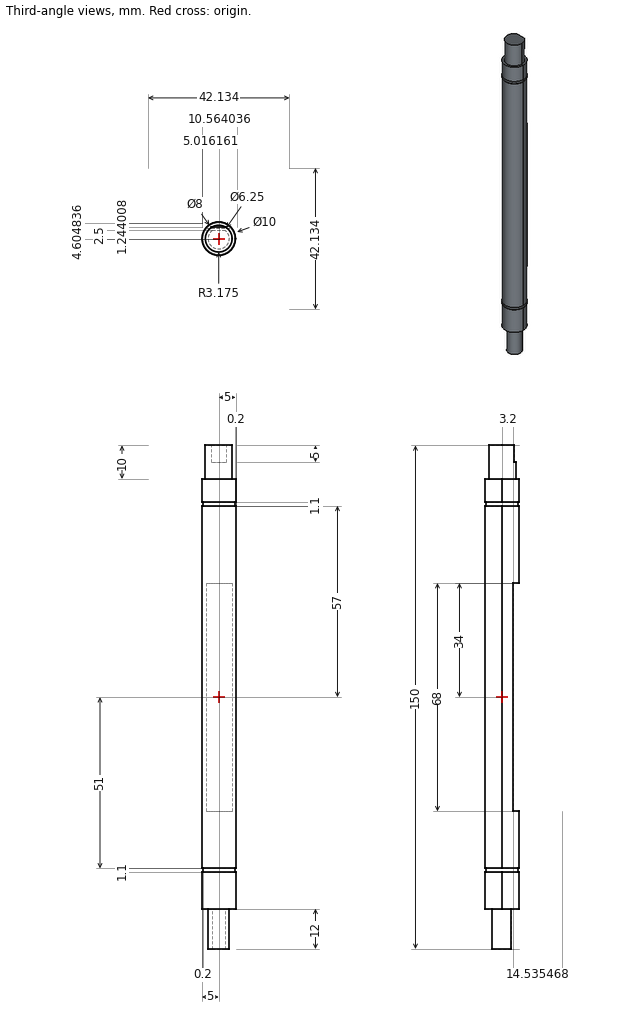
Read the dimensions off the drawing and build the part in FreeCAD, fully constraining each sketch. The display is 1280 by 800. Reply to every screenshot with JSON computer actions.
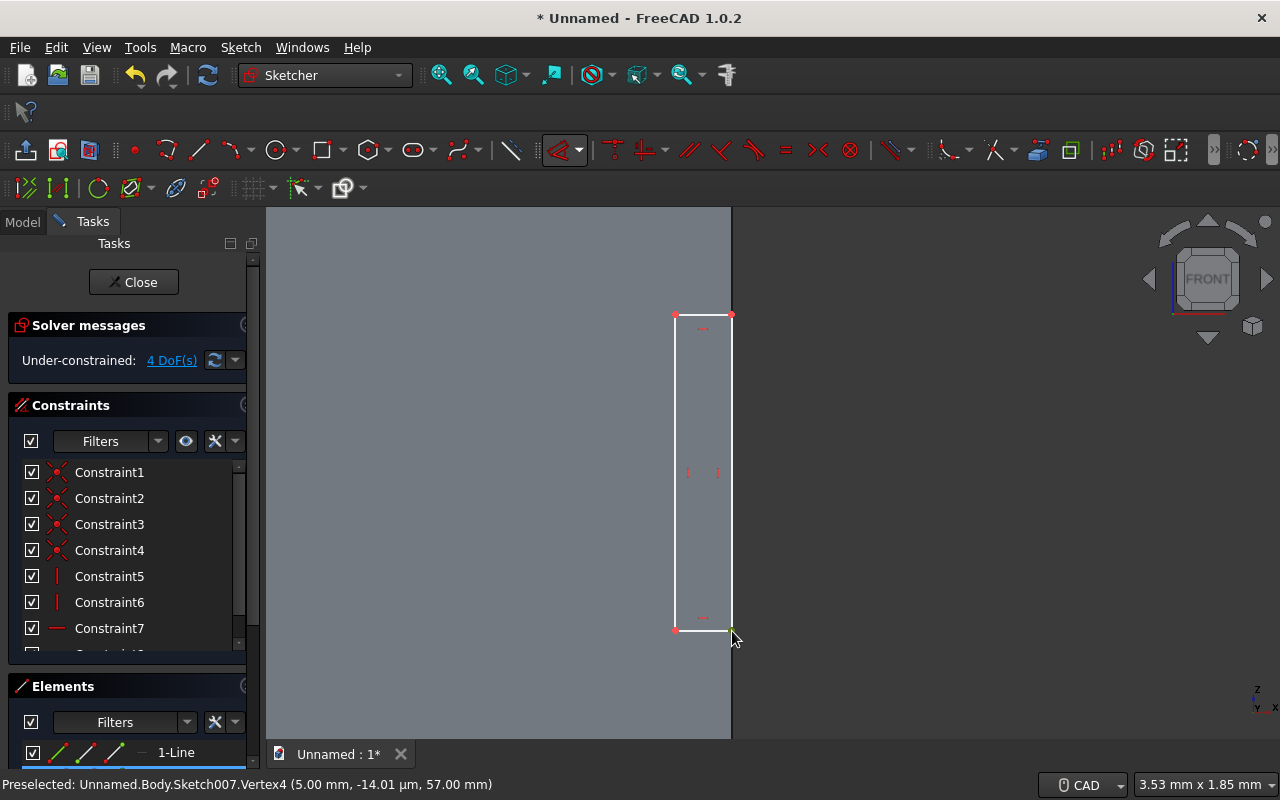
{"action": "key", "text": "l"}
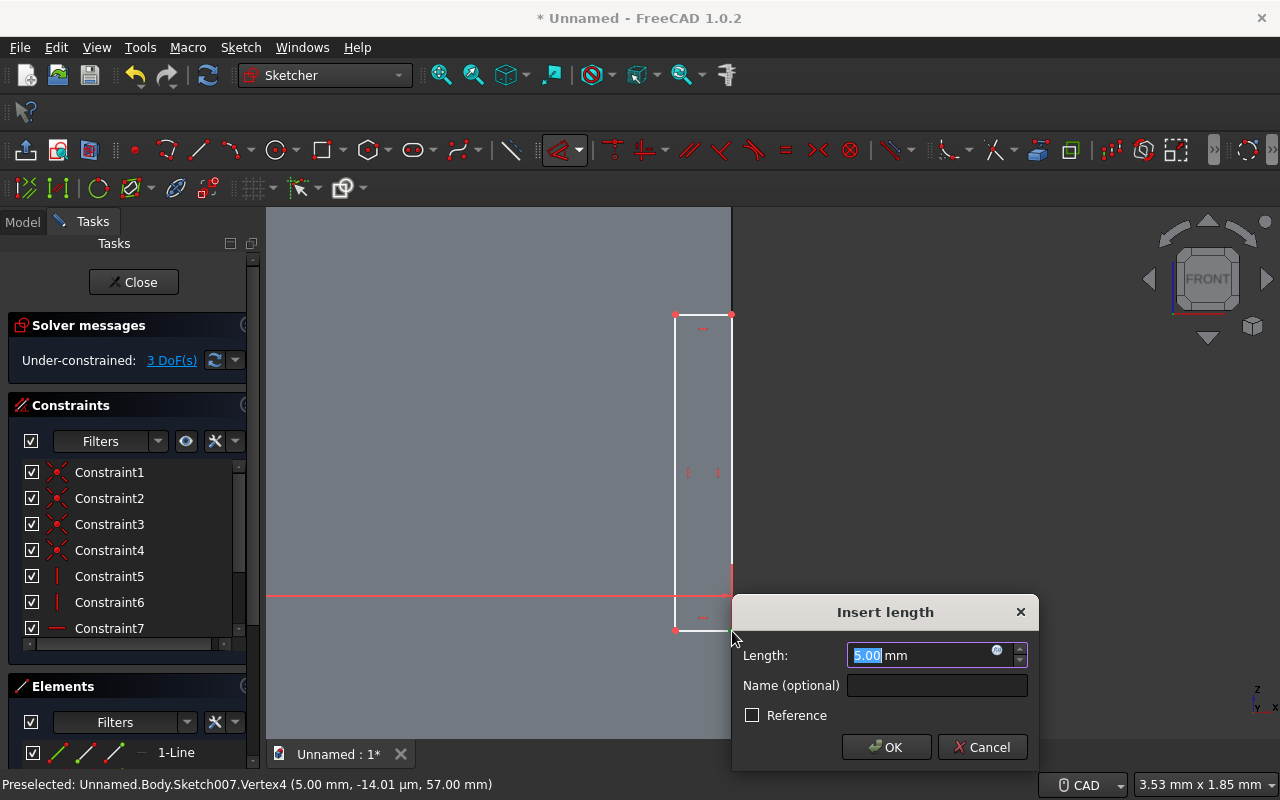
{"action": "type", "text": "5"}
{"action": "key", "text": "Return"}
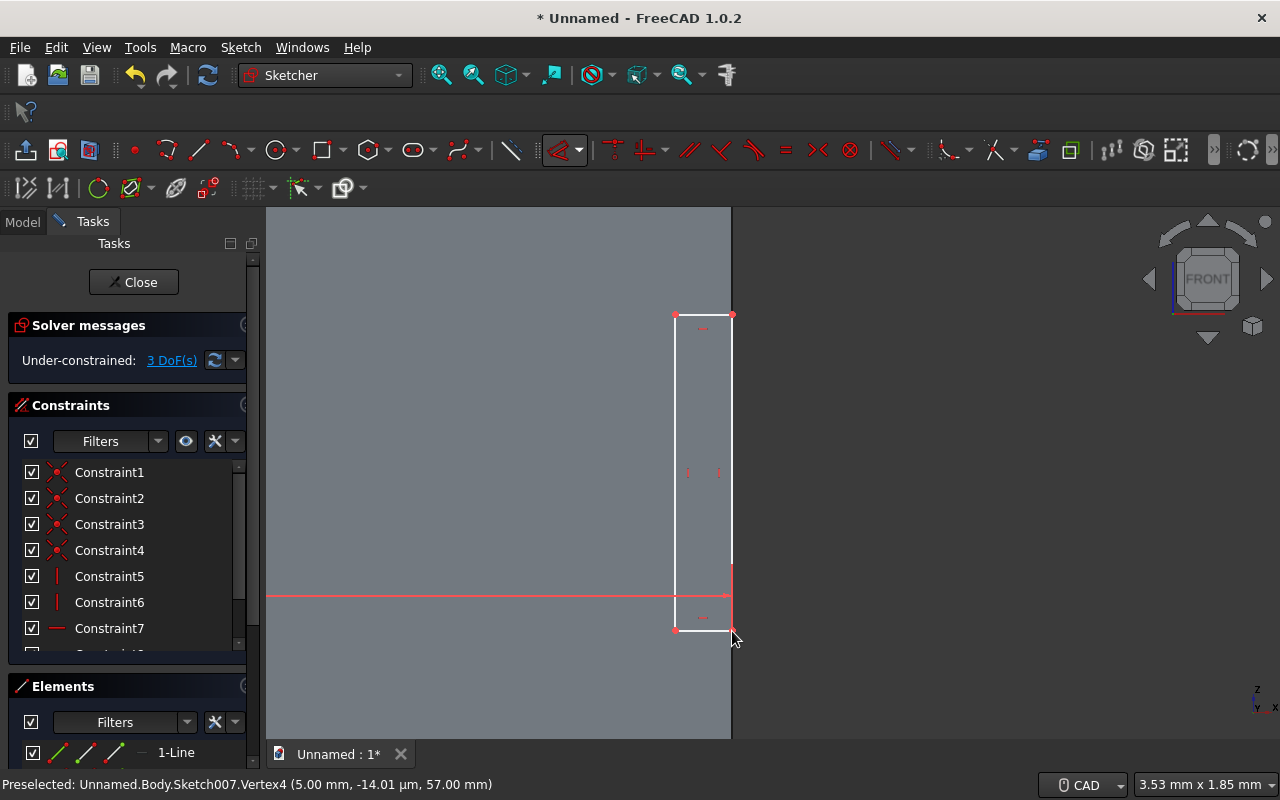
{"action": "left_click", "coordinate": [675, 410]}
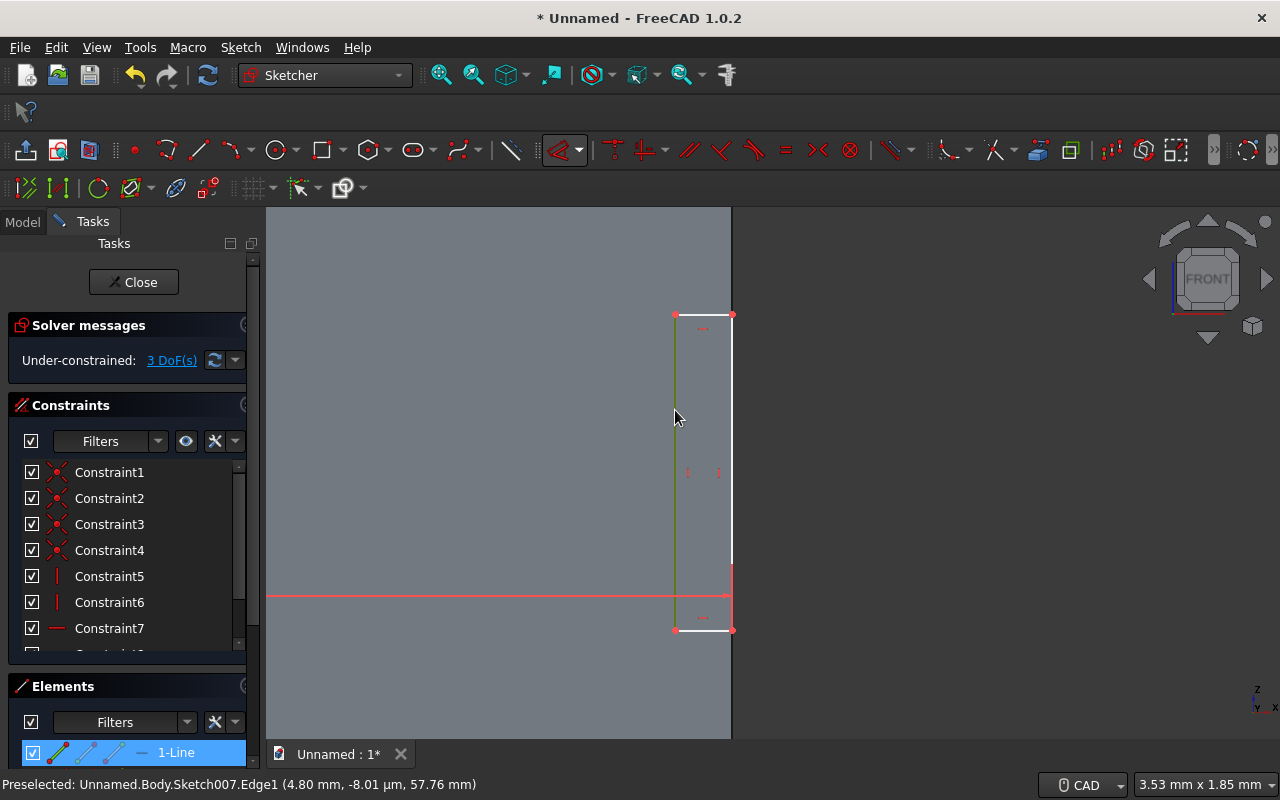
{"action": "key", "text": "i"}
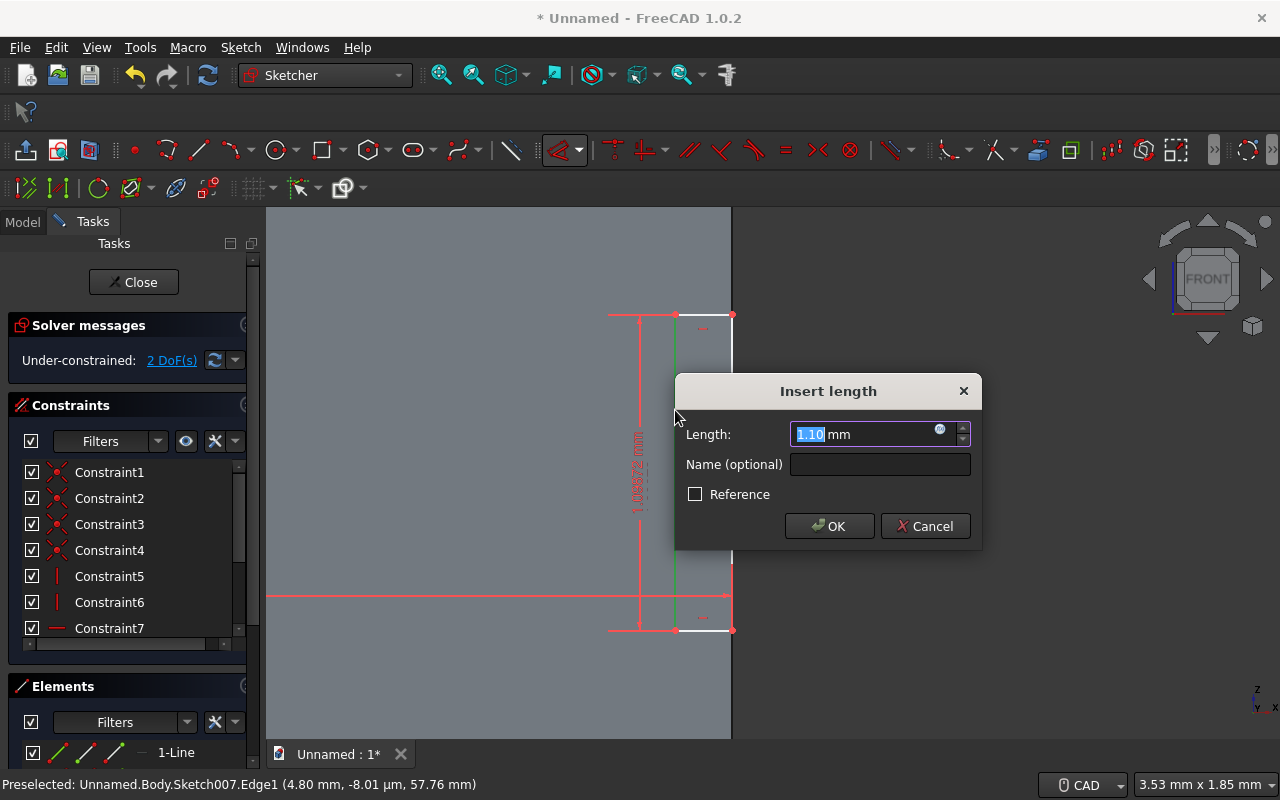
{"action": "type", "text": "1.1"}
{"action": "key", "text": "Return"}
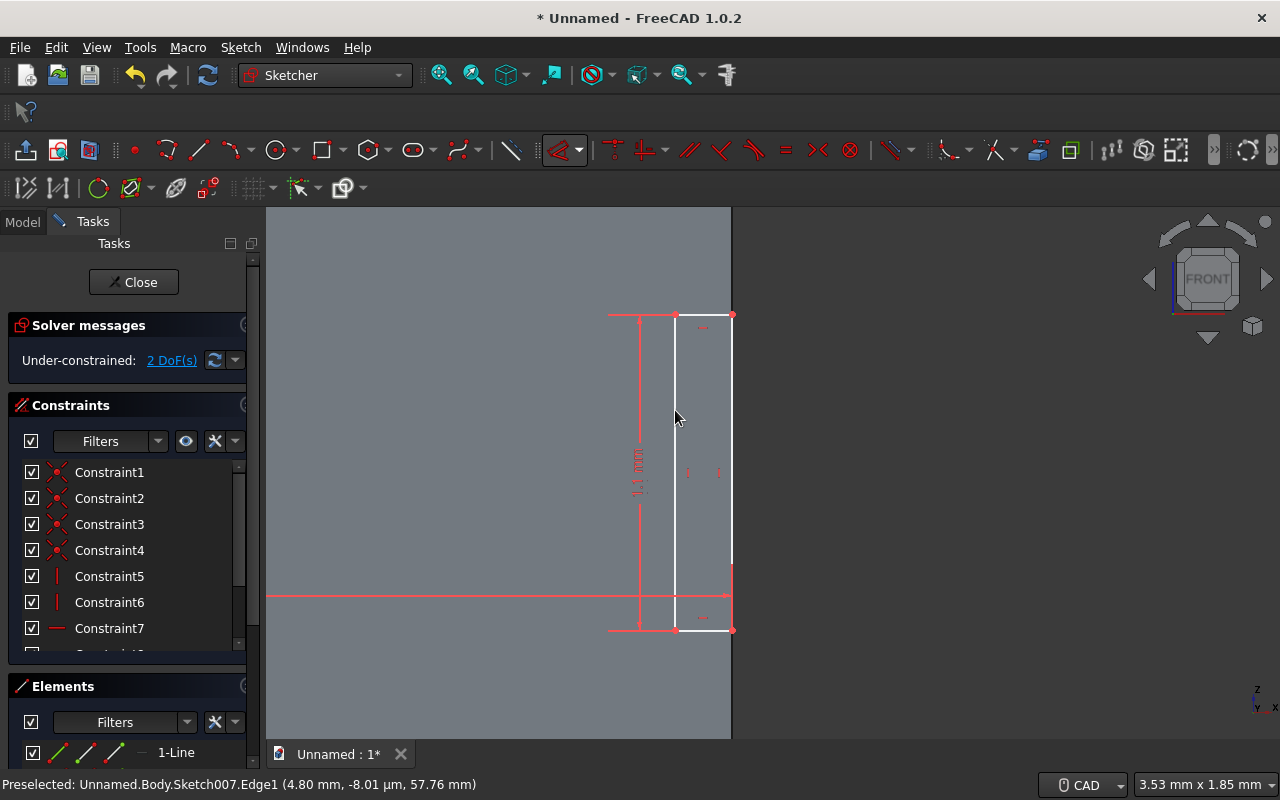
{"action": "left_click", "coordinate": [692, 631]}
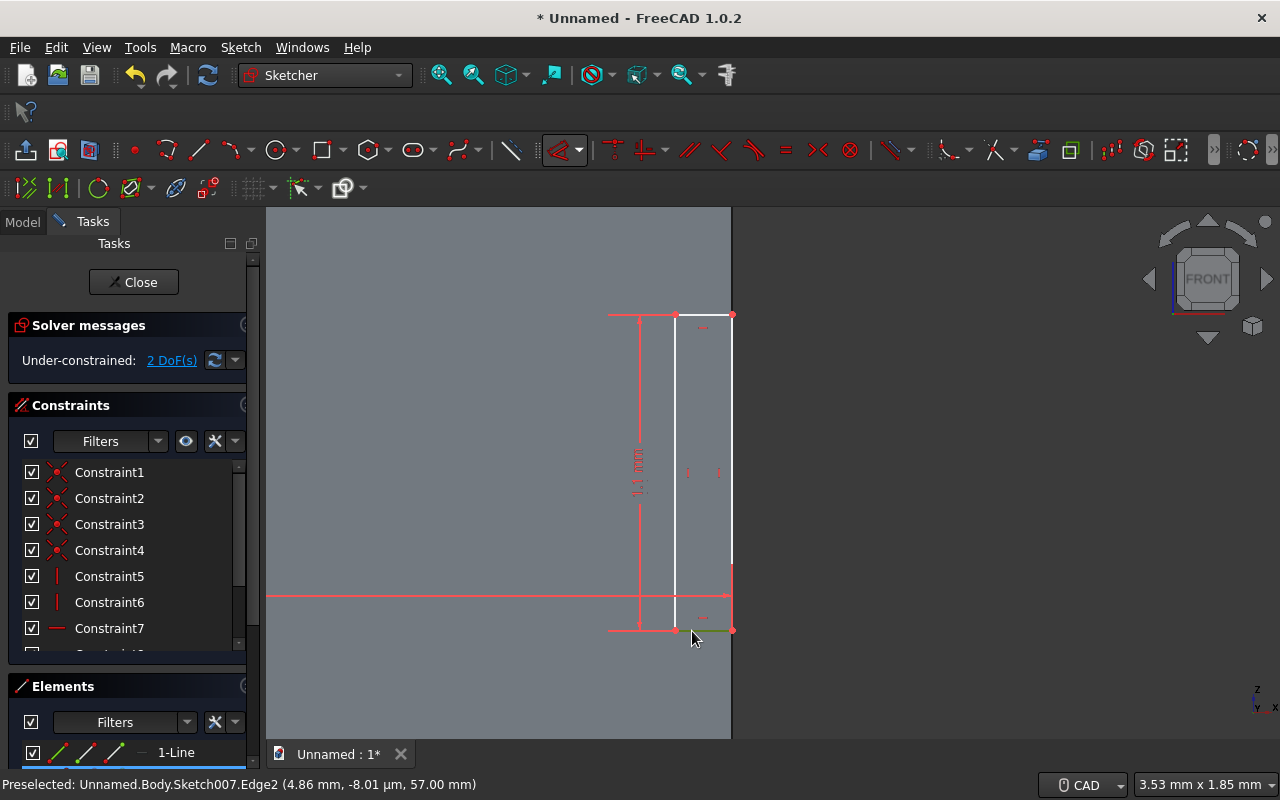
{"action": "key", "text": "l"}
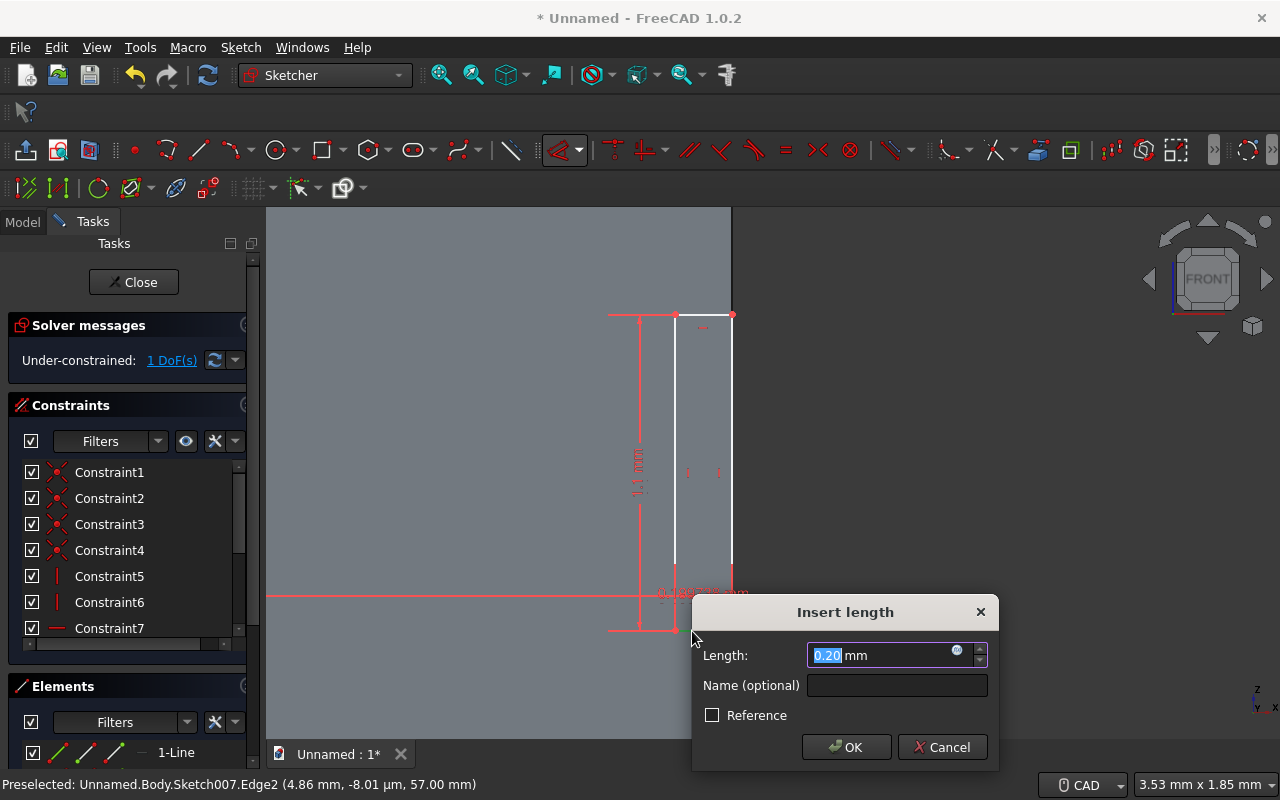
{"action": "type", "text": "0.2"}
{"action": "key", "text": "Return"}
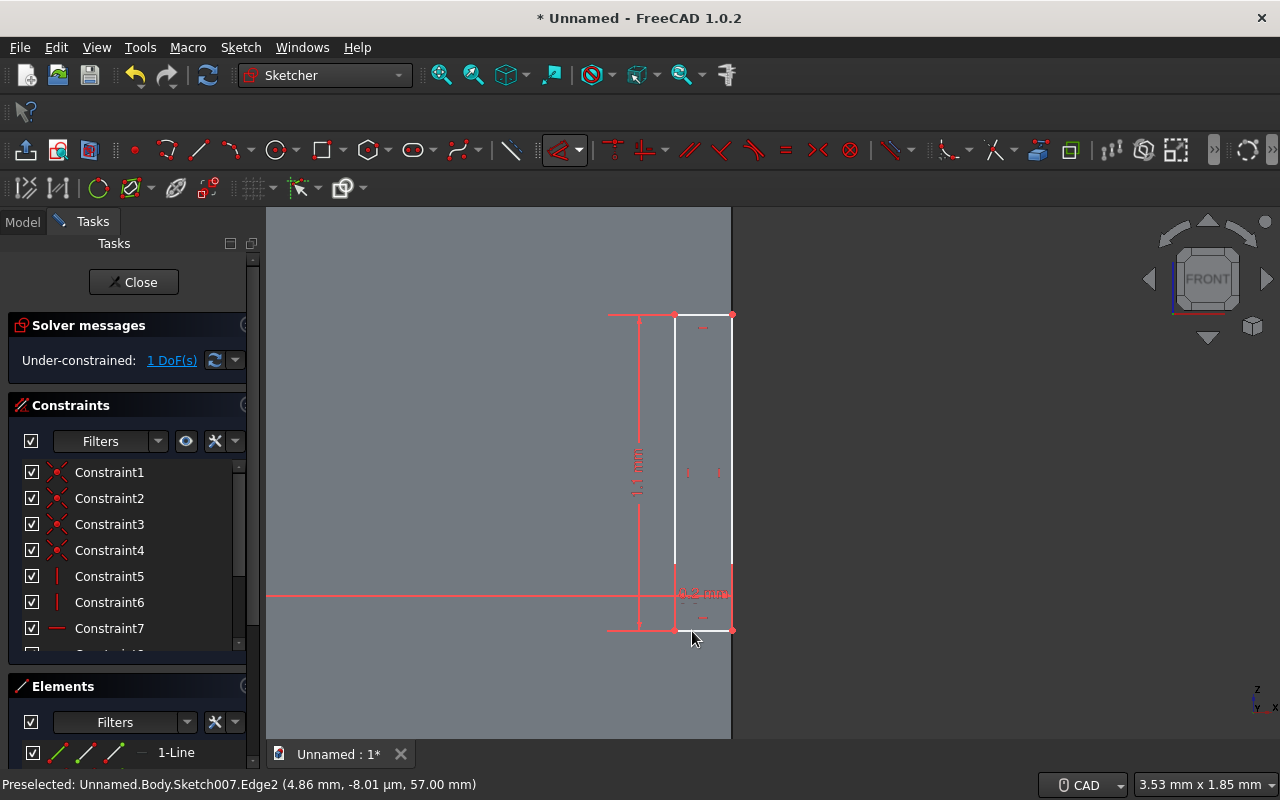
{"action": "left_click", "coordinate": [675, 631]}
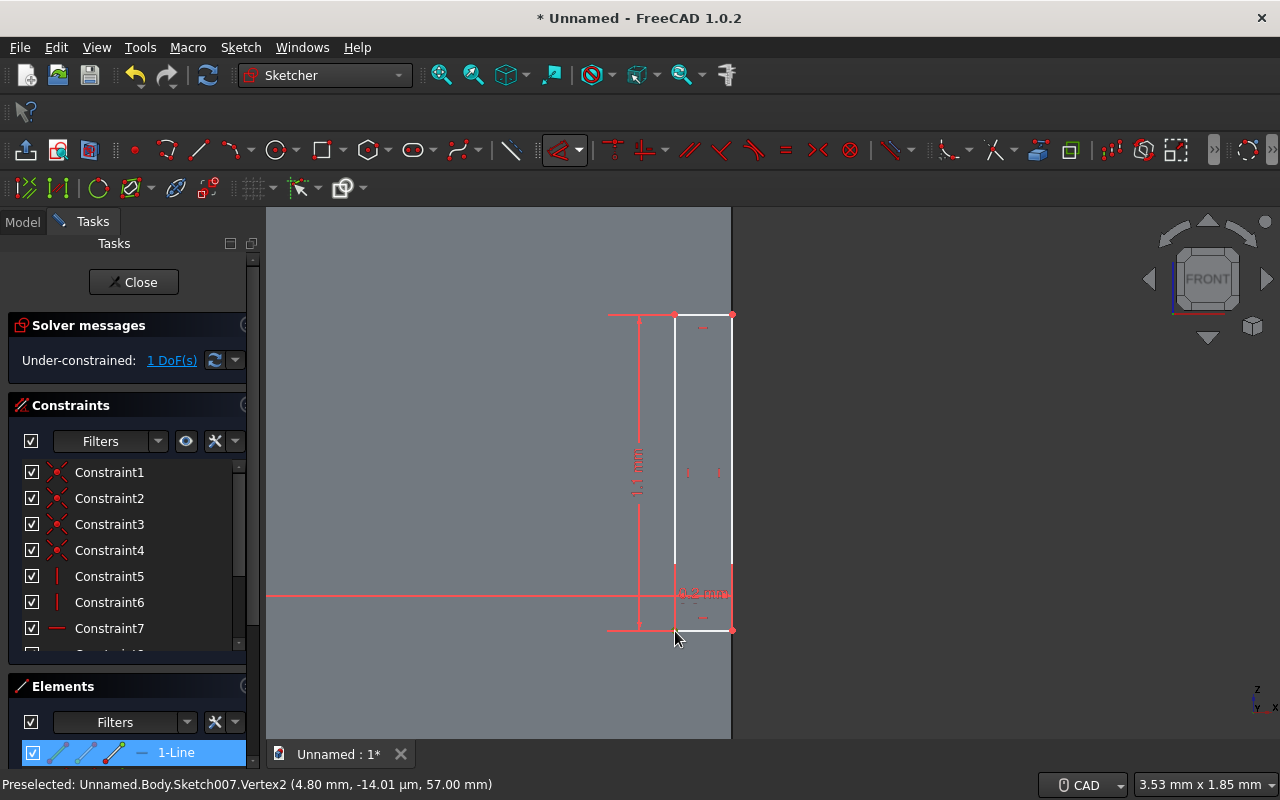
{"action": "key", "text": "i"}